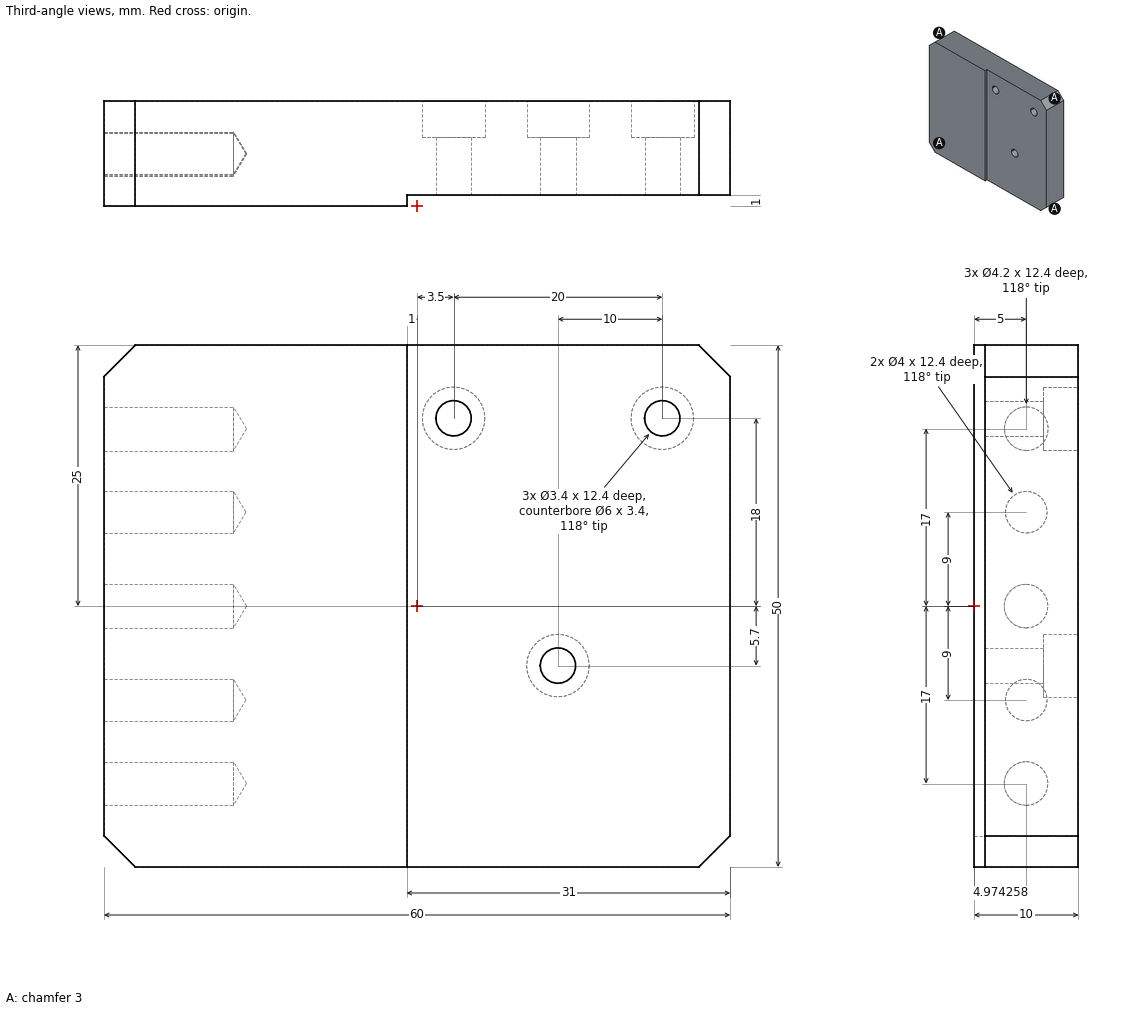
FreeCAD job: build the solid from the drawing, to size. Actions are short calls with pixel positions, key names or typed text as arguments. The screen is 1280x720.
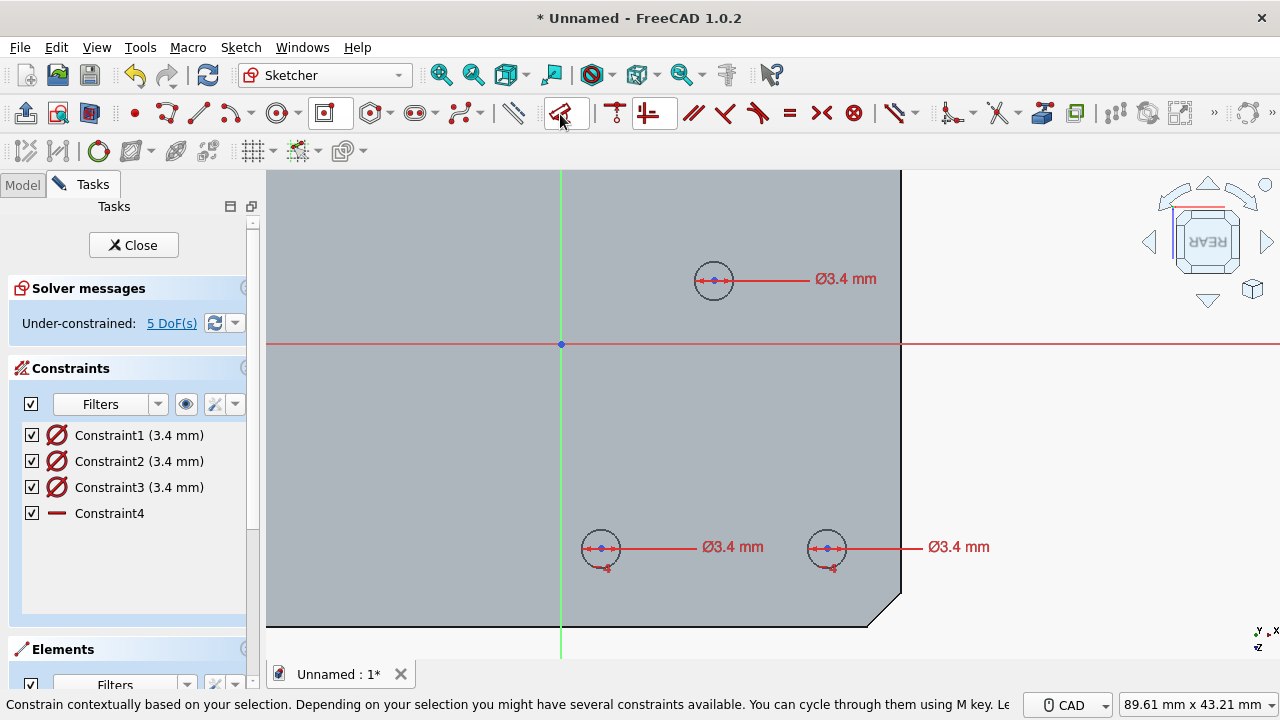
click(827, 549)
click(527, 447)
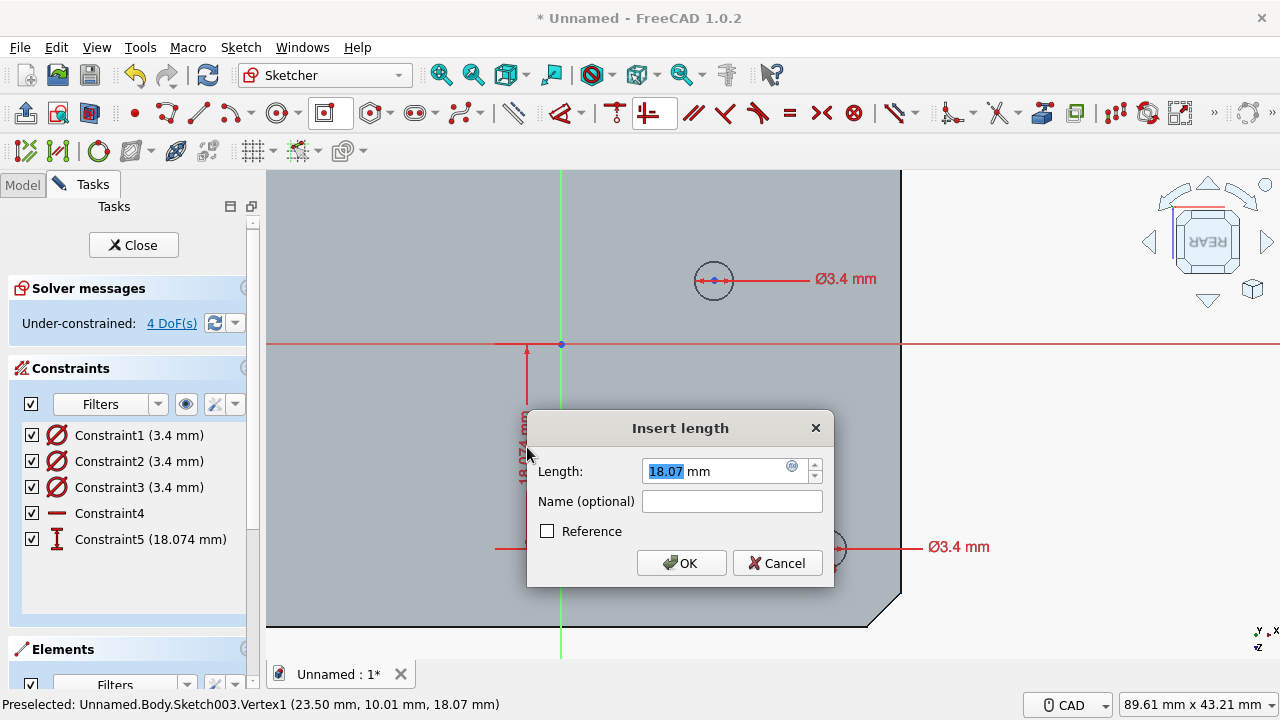
text(18)
key(Return)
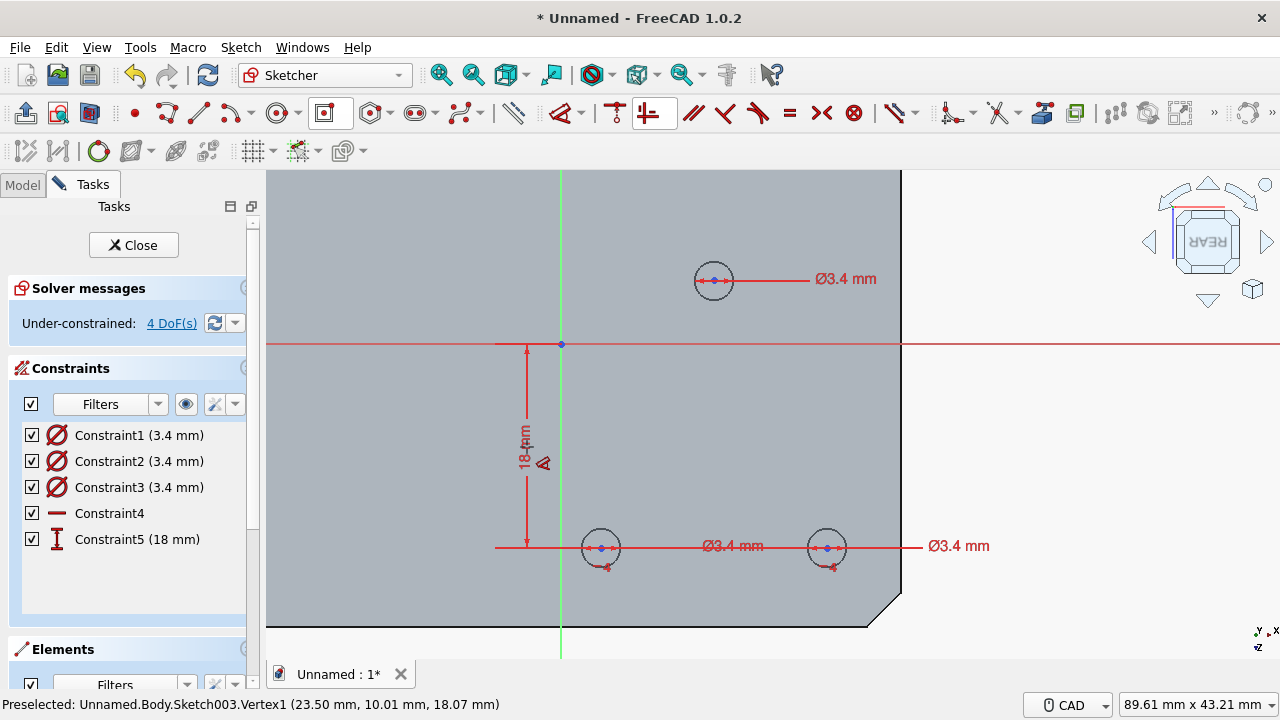
click(601, 548)
click(581, 582)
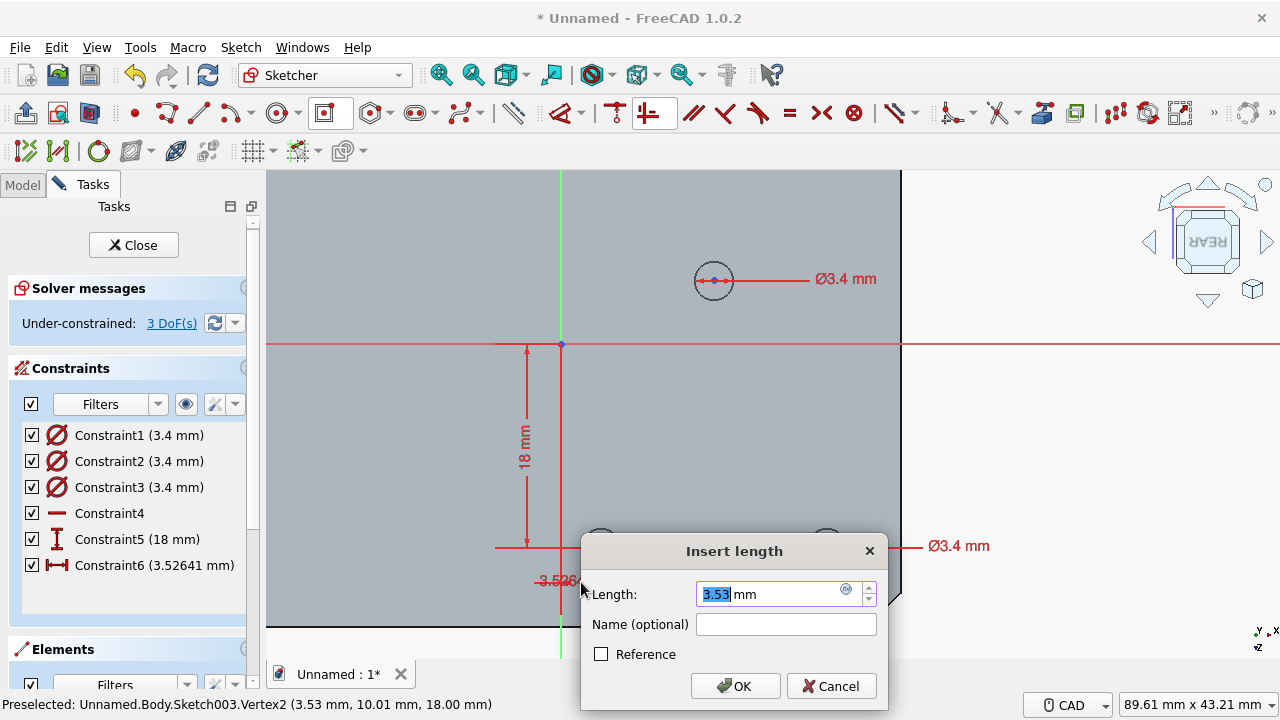
text(3.5)
key(Return)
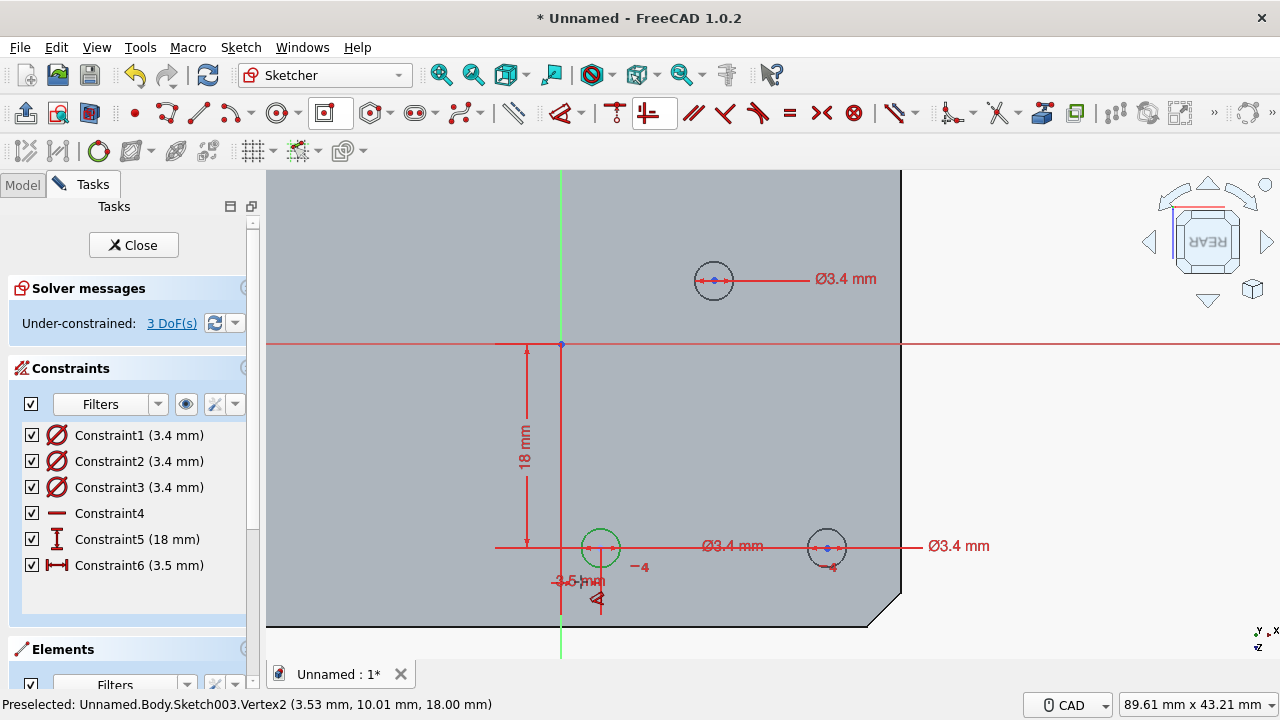
click(714, 281)
click(527, 313)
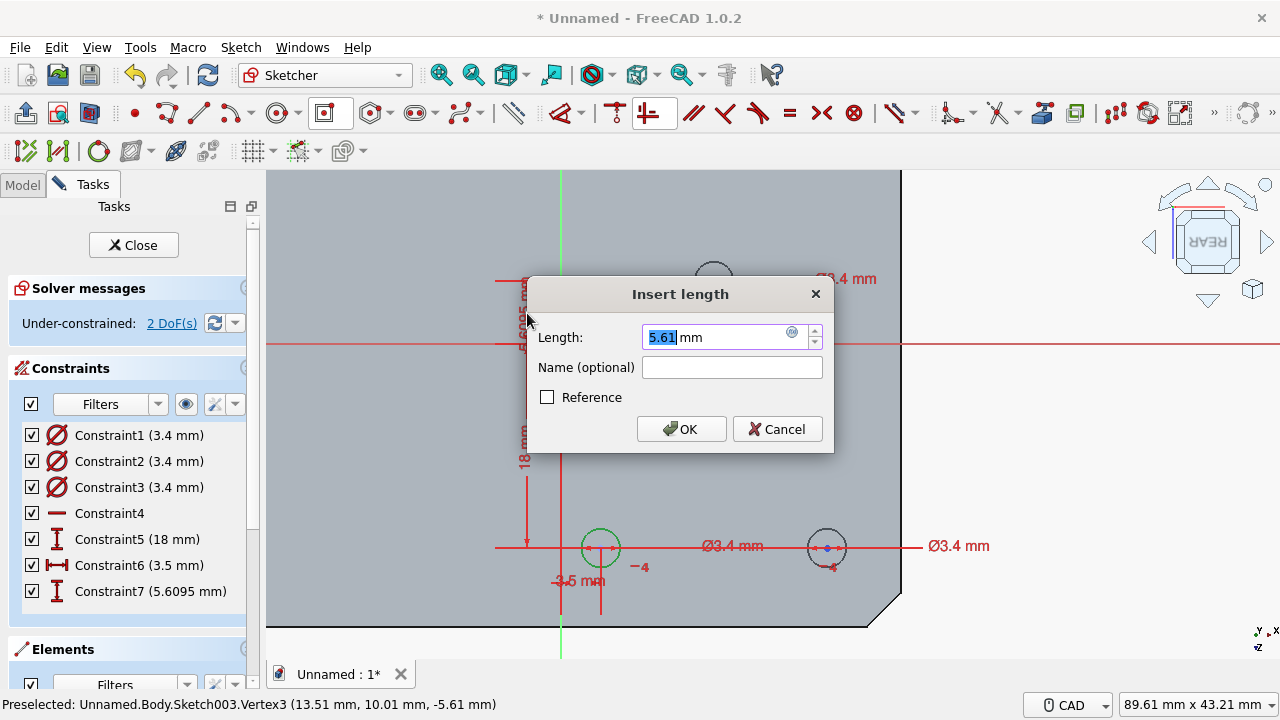
text(5.7)
key(Return)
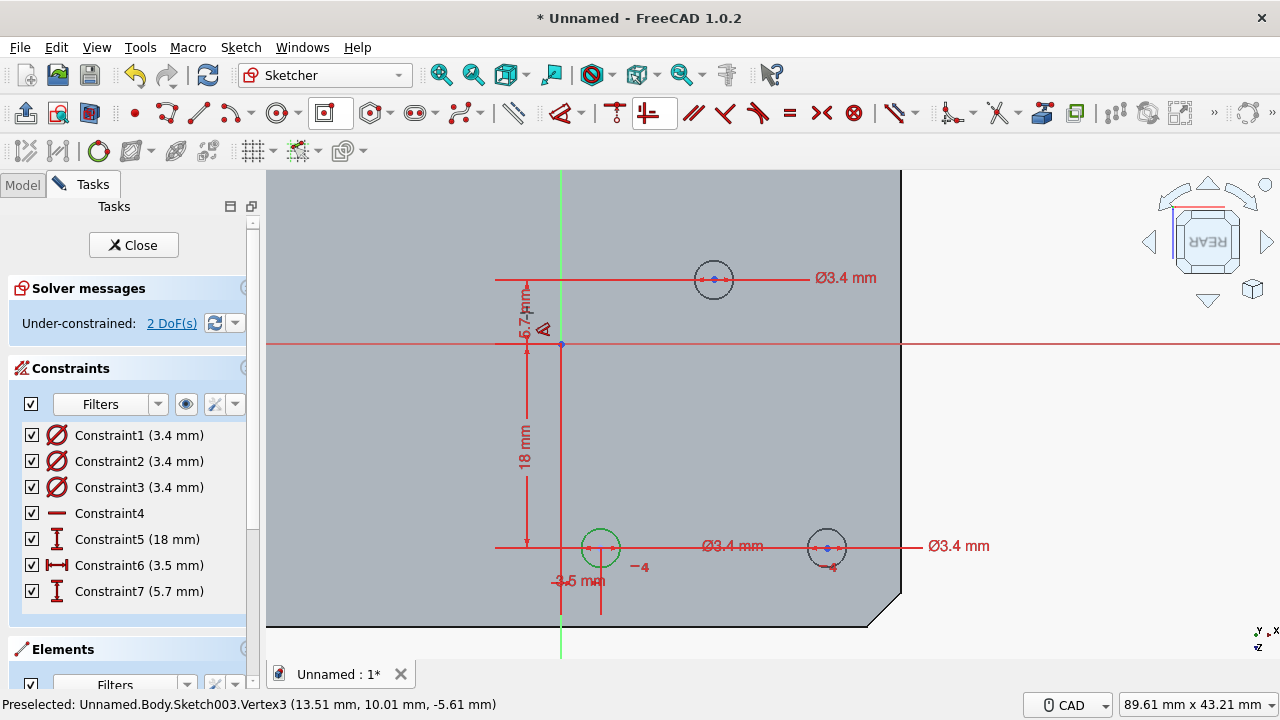
click(827, 548)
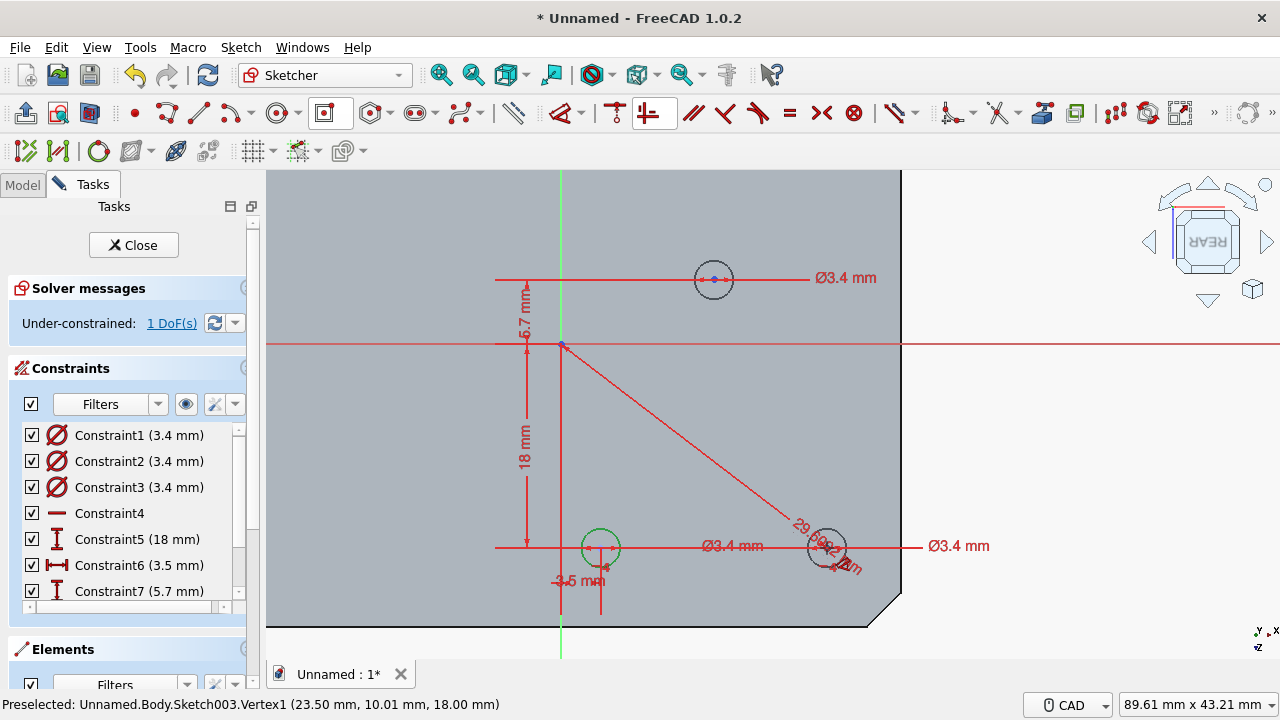
click(601, 548)
click(714, 582)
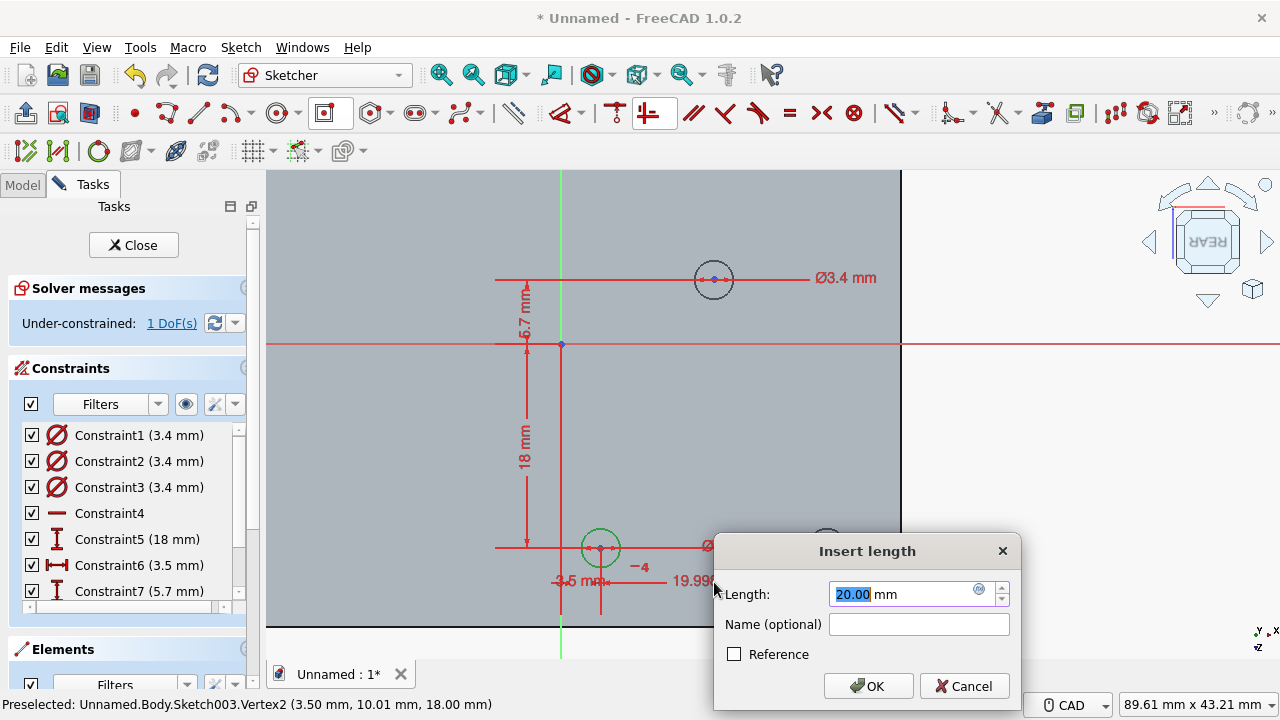
text(20)
key(Return)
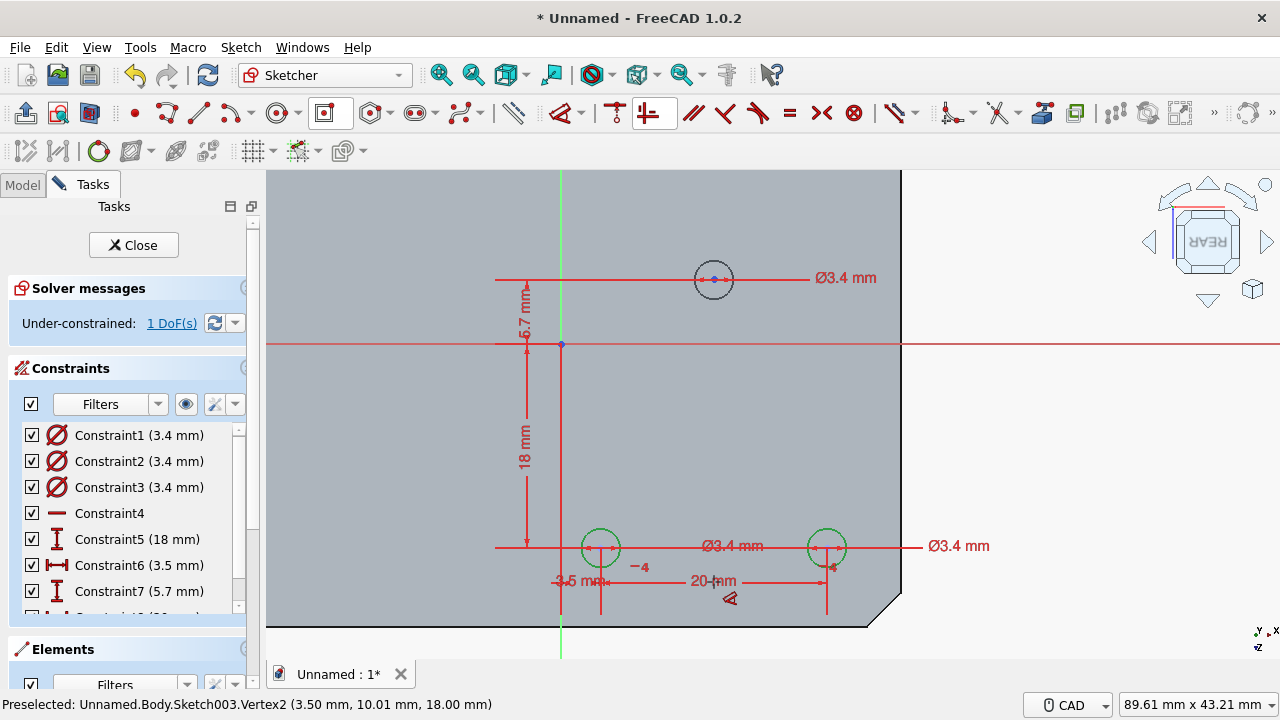
click(827, 548)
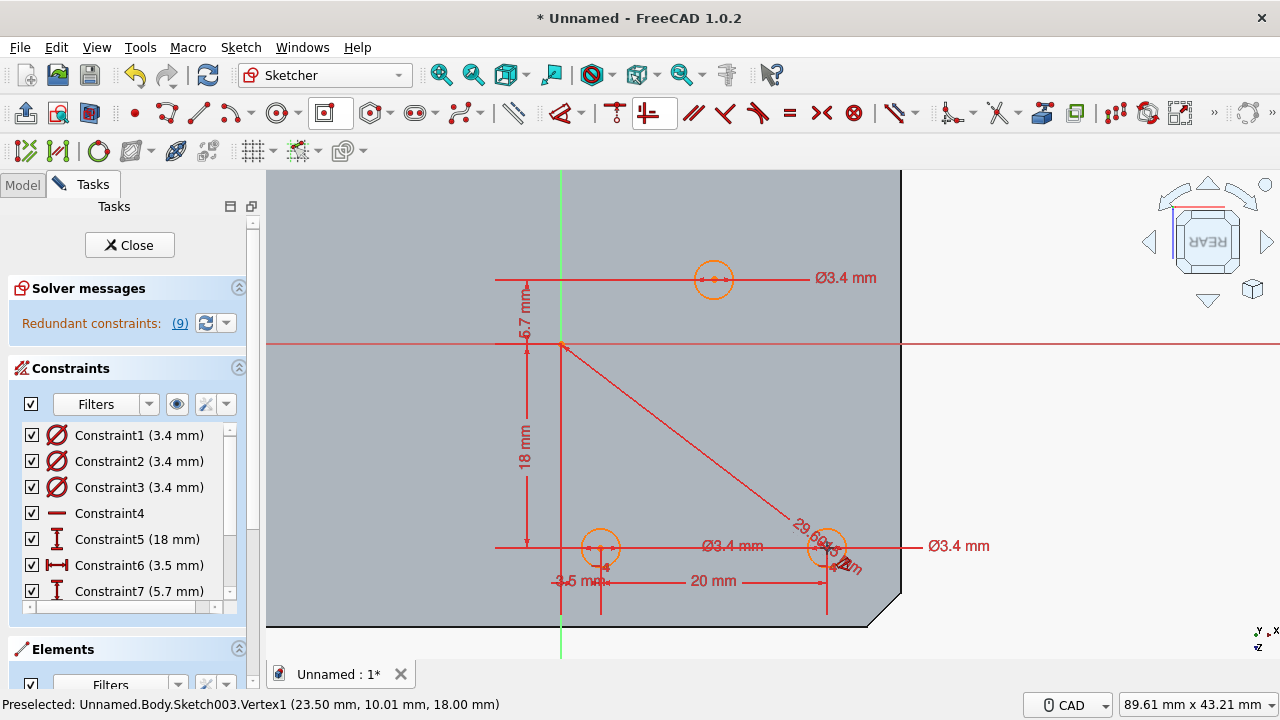
click(714, 280)
click(797, 582)